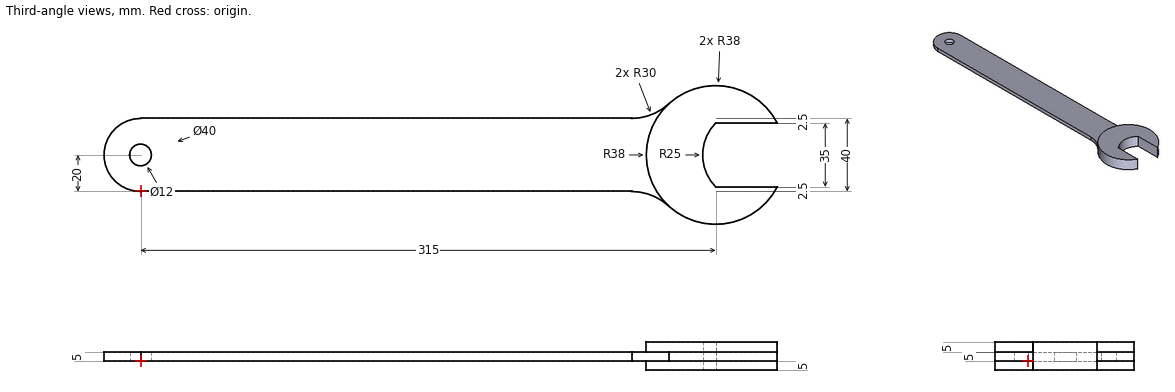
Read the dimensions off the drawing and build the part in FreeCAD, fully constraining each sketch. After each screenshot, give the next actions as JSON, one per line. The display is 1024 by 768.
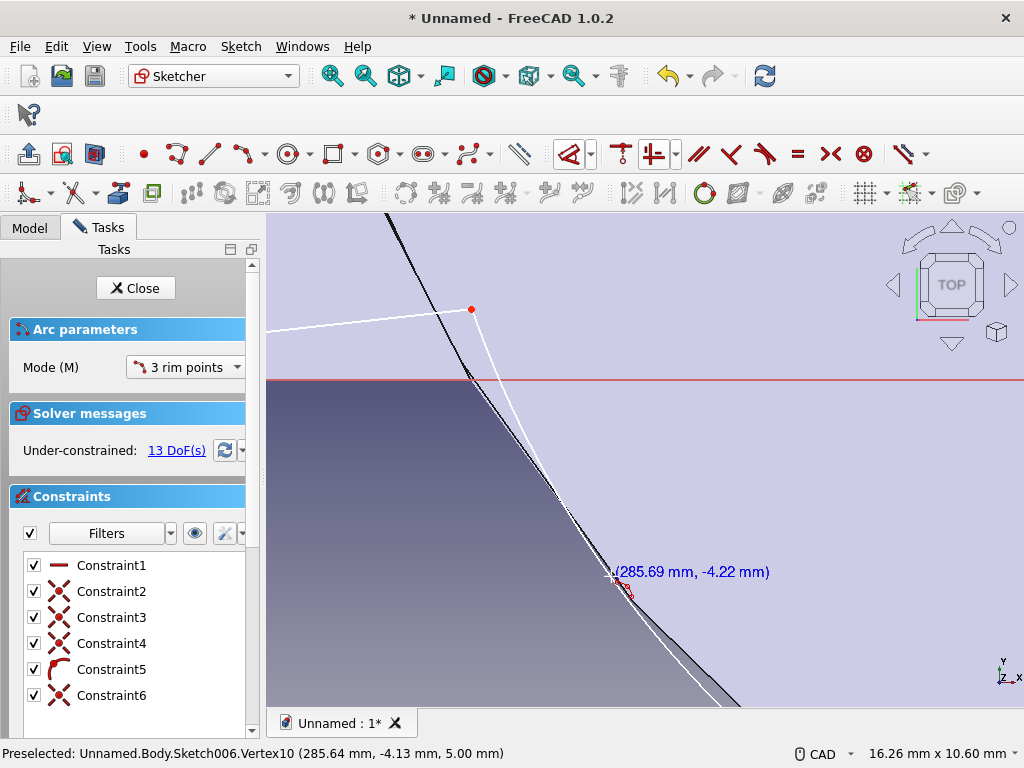
{"action": "scroll", "coordinate": [611, 586], "scroll_direction": "down", "scroll_amount": 11}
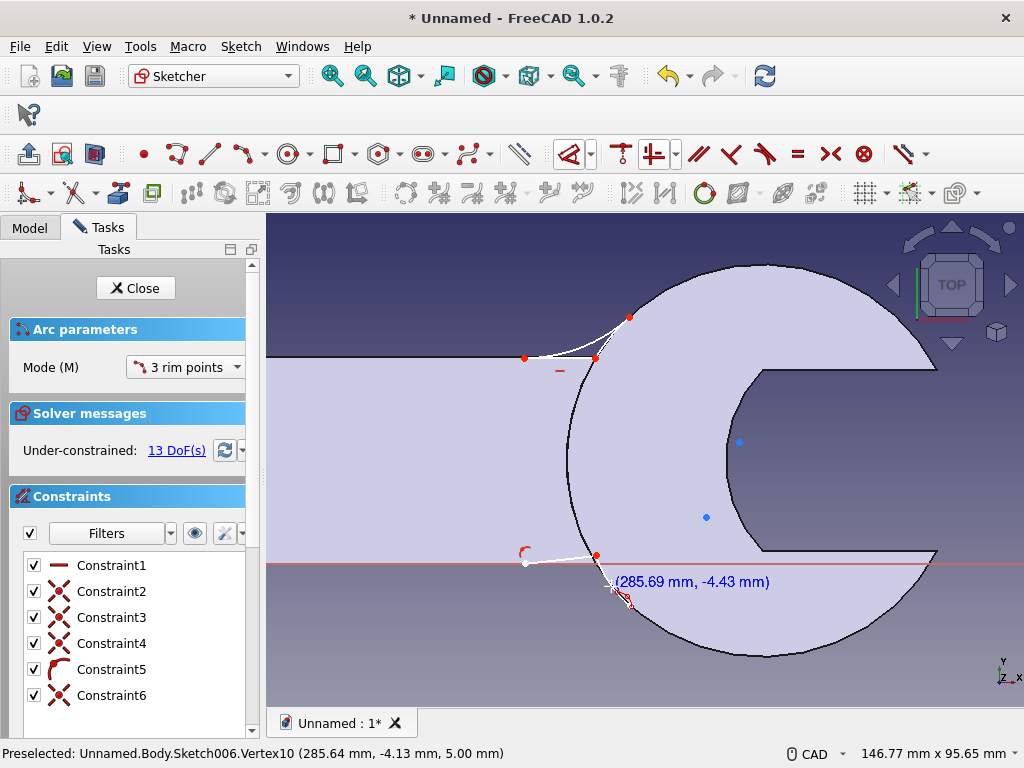
{"action": "left_click", "coordinate": [630, 606]}
{"action": "left_click", "coordinate": [525, 564]}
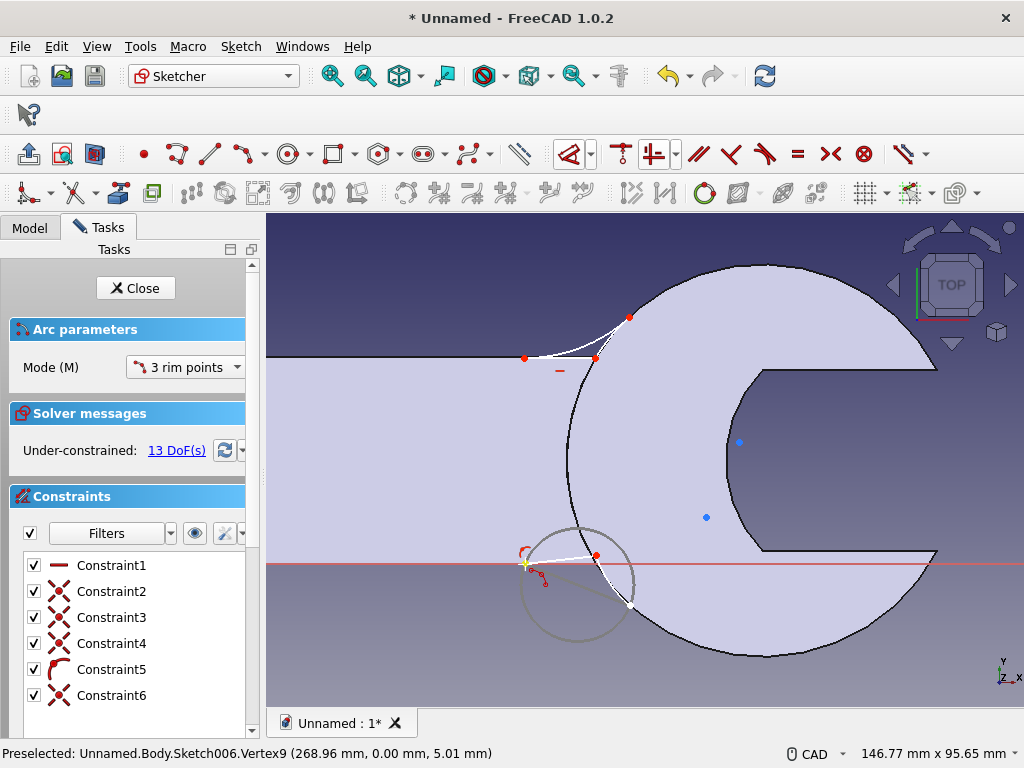
{"action": "scroll", "coordinate": [581, 575], "scroll_direction": "up", "scroll_amount": 3}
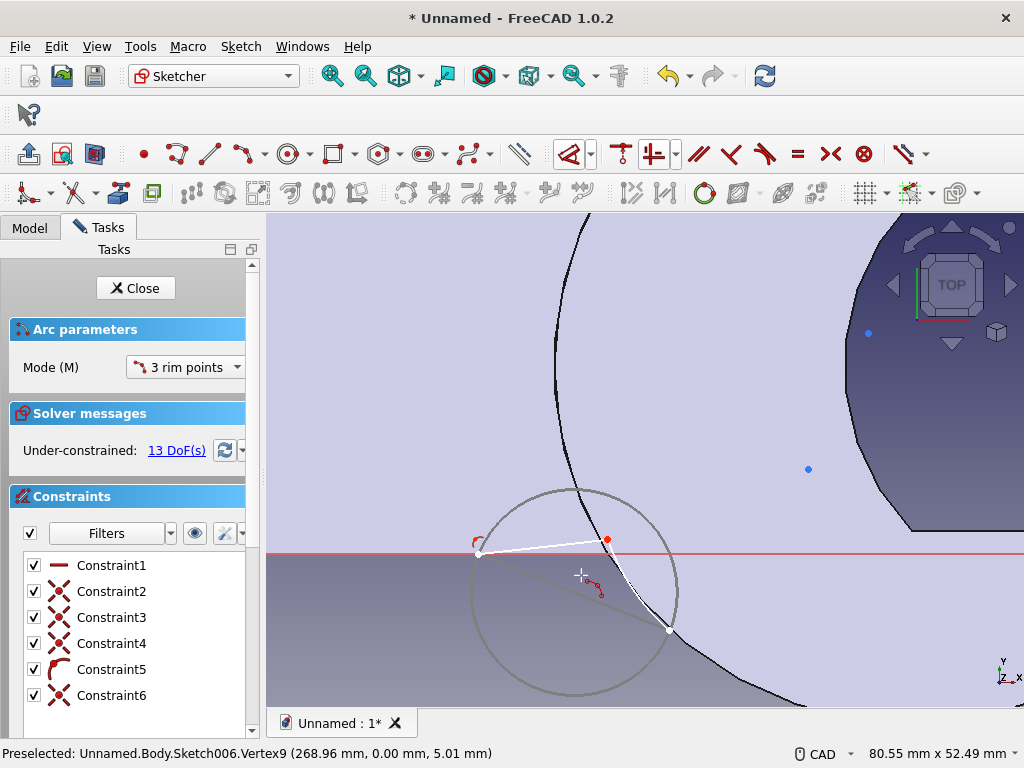
{"action": "left_click", "coordinate": [581, 574]}
{"action": "key", "text": "Escape"}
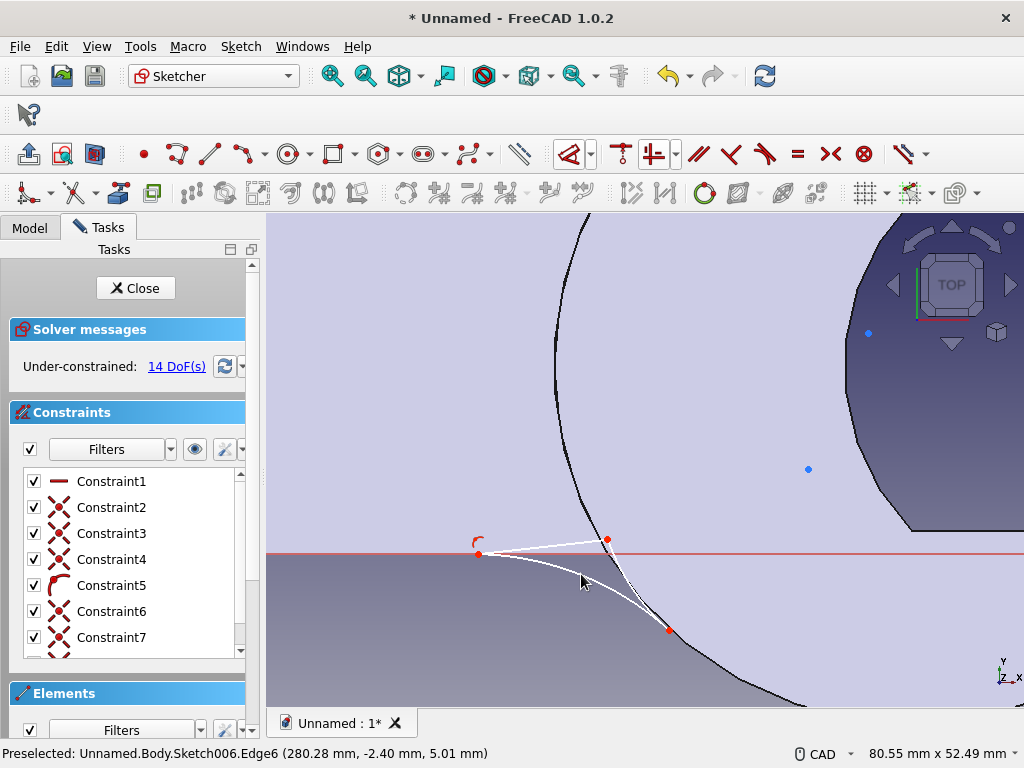
{"action": "scroll", "coordinate": [580, 574], "scroll_direction": "down", "scroll_amount": 3}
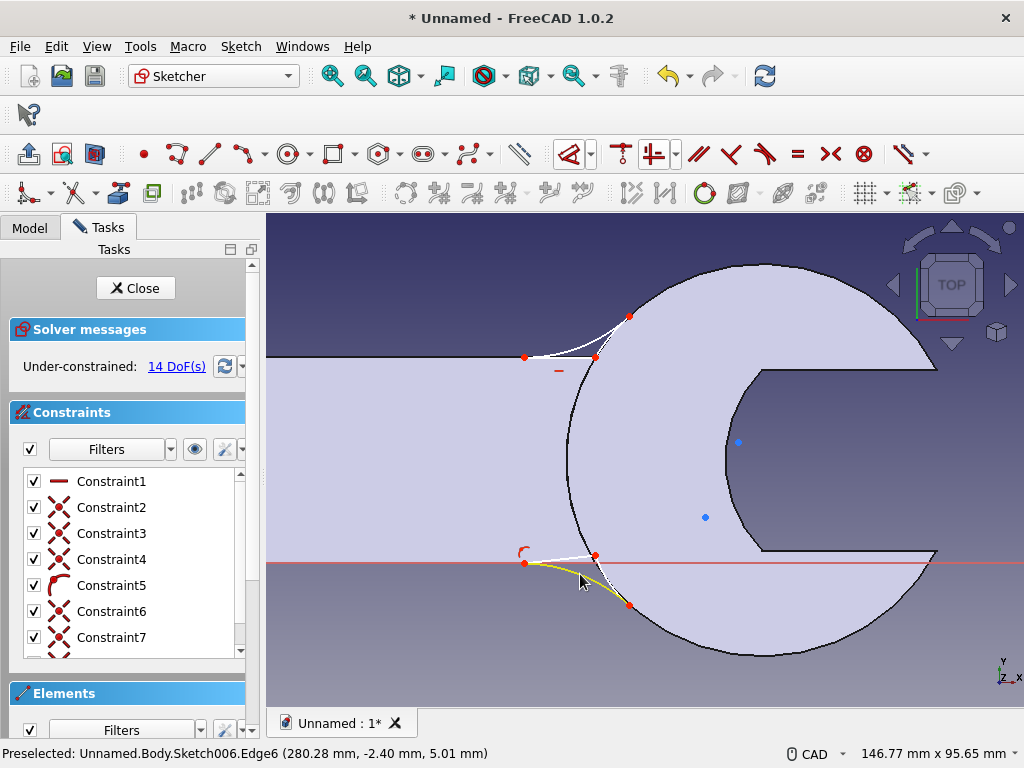
{"action": "scroll", "coordinate": [574, 358], "scroll_direction": "up", "scroll_amount": 3}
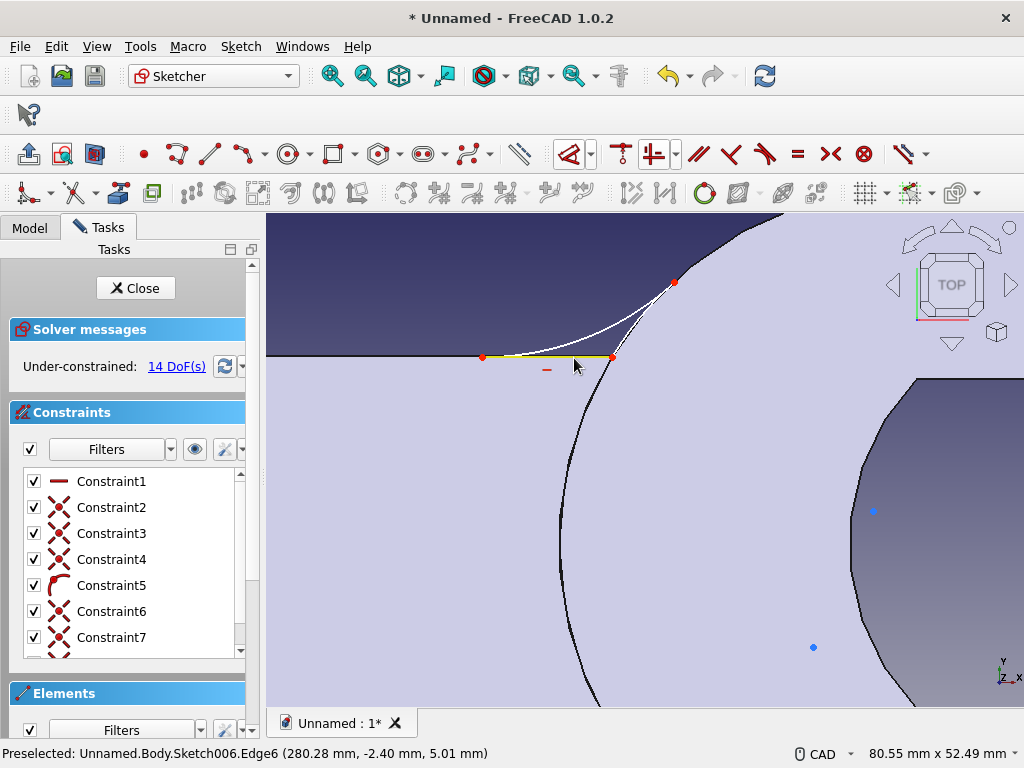
{"action": "left_click", "coordinate": [573, 357]}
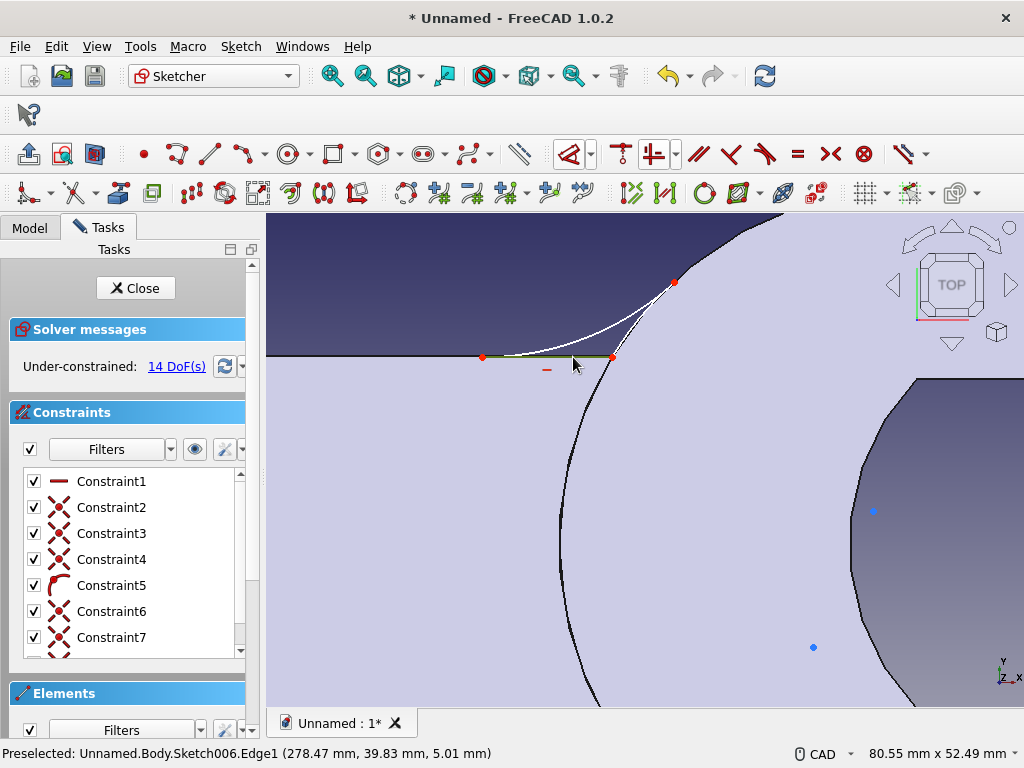
{"action": "left_click", "coordinate": [623, 320]}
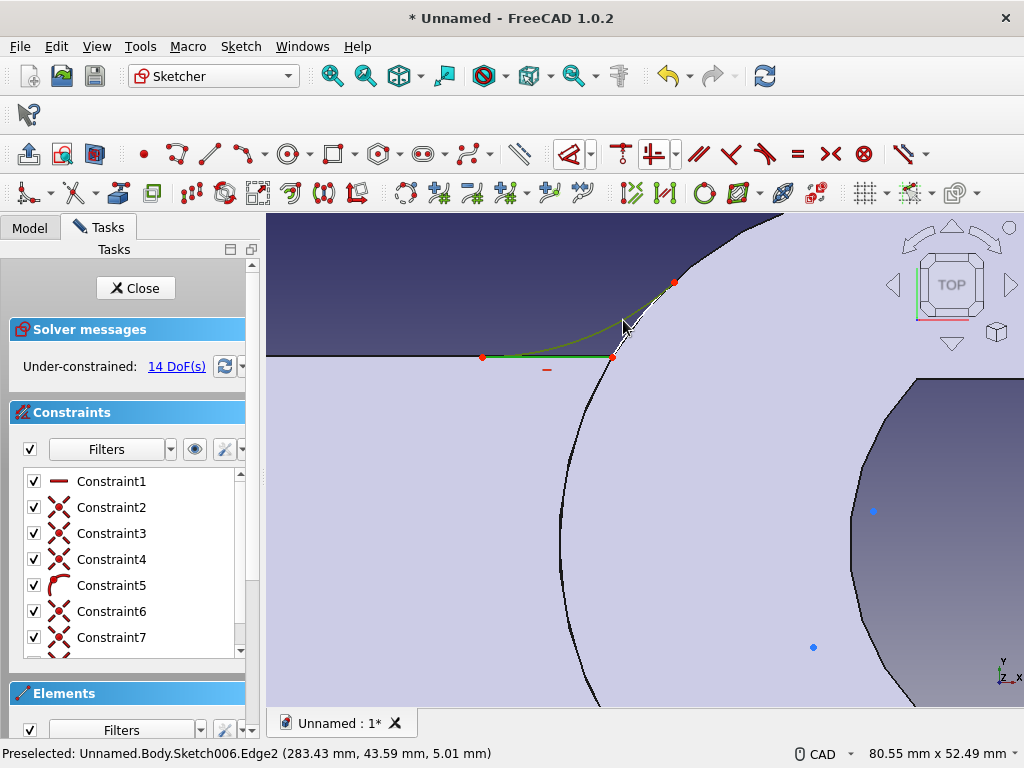
{"action": "left_click", "coordinate": [765, 154]}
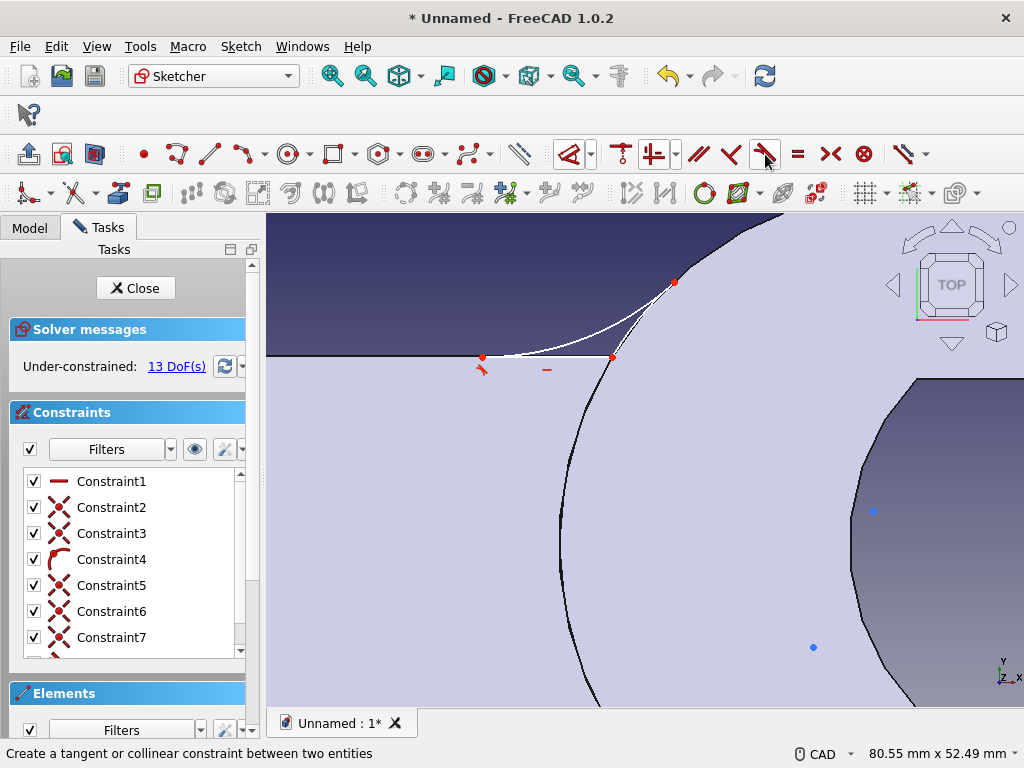
{"action": "left_click", "coordinate": [623, 320]}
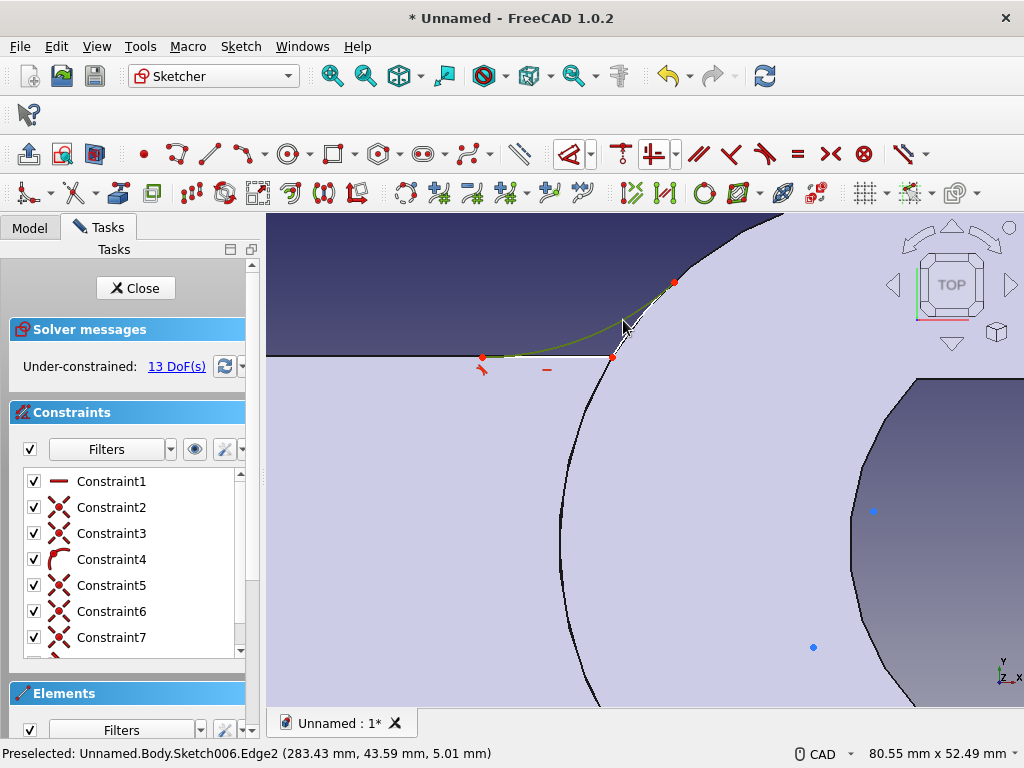
{"action": "left_click", "coordinate": [628, 333]}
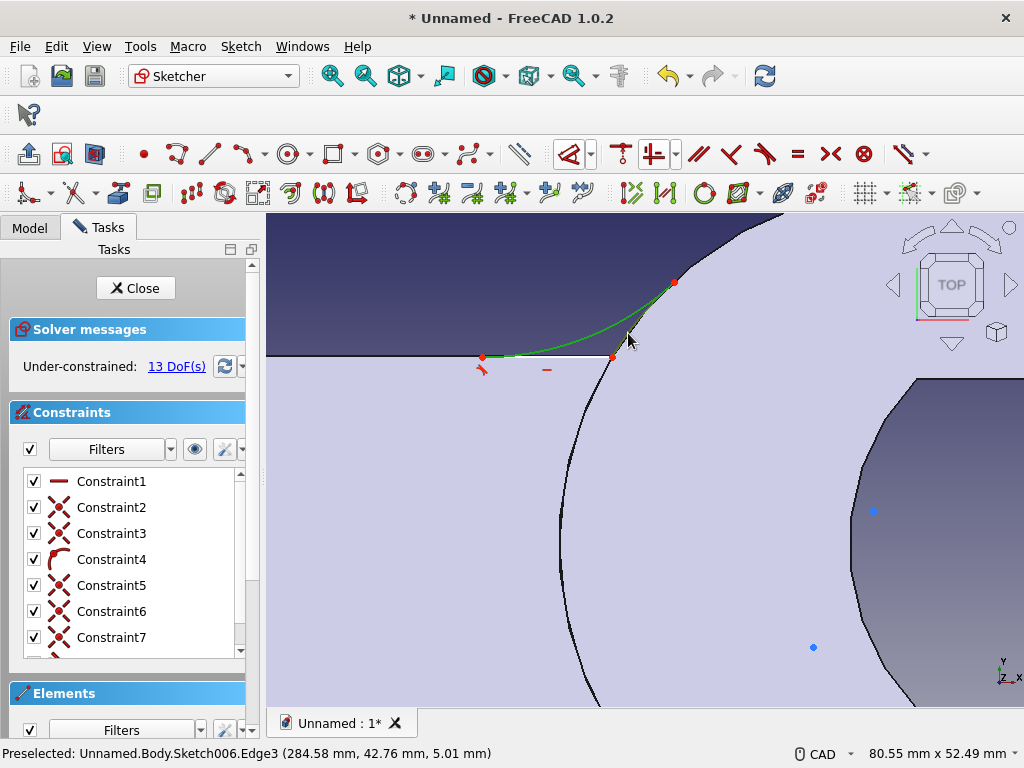
{"action": "left_click", "coordinate": [765, 154]}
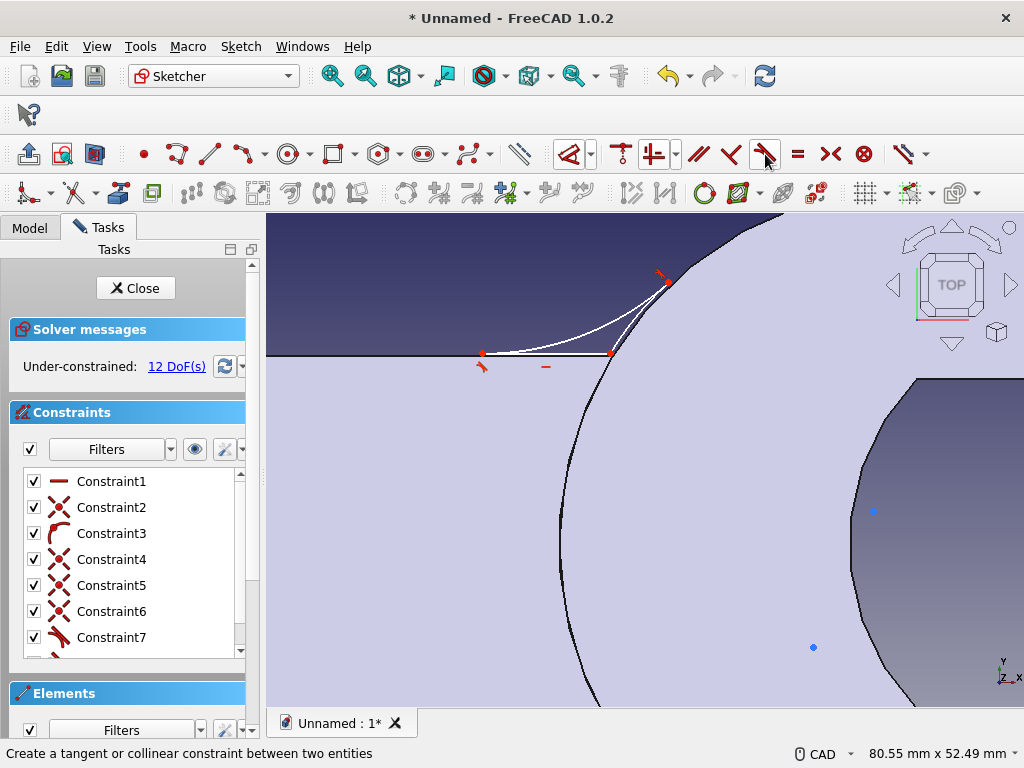
{"action": "scroll", "coordinate": [574, 358], "scroll_direction": "down", "scroll_amount": 3}